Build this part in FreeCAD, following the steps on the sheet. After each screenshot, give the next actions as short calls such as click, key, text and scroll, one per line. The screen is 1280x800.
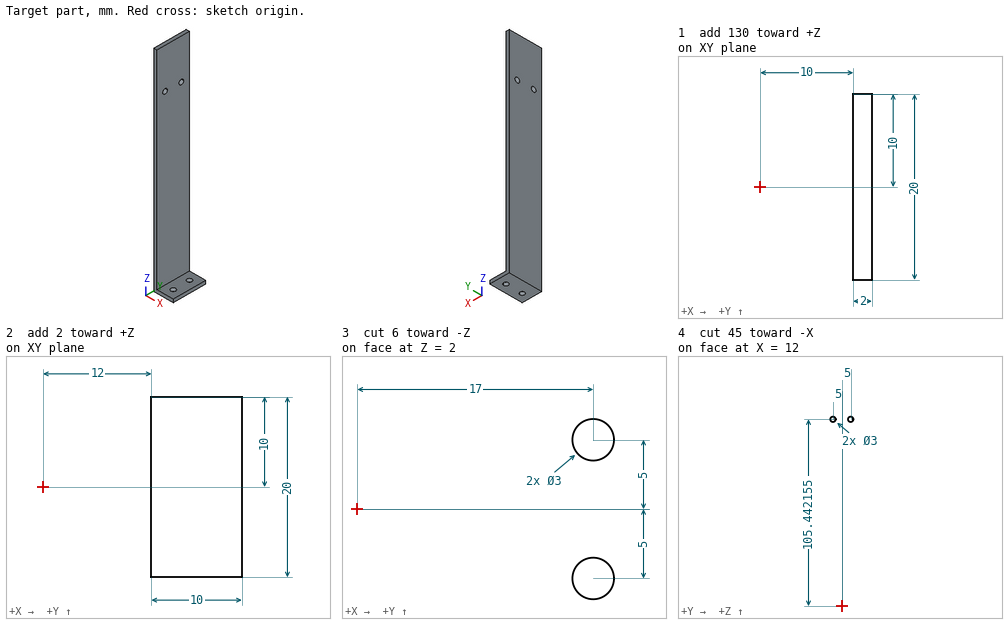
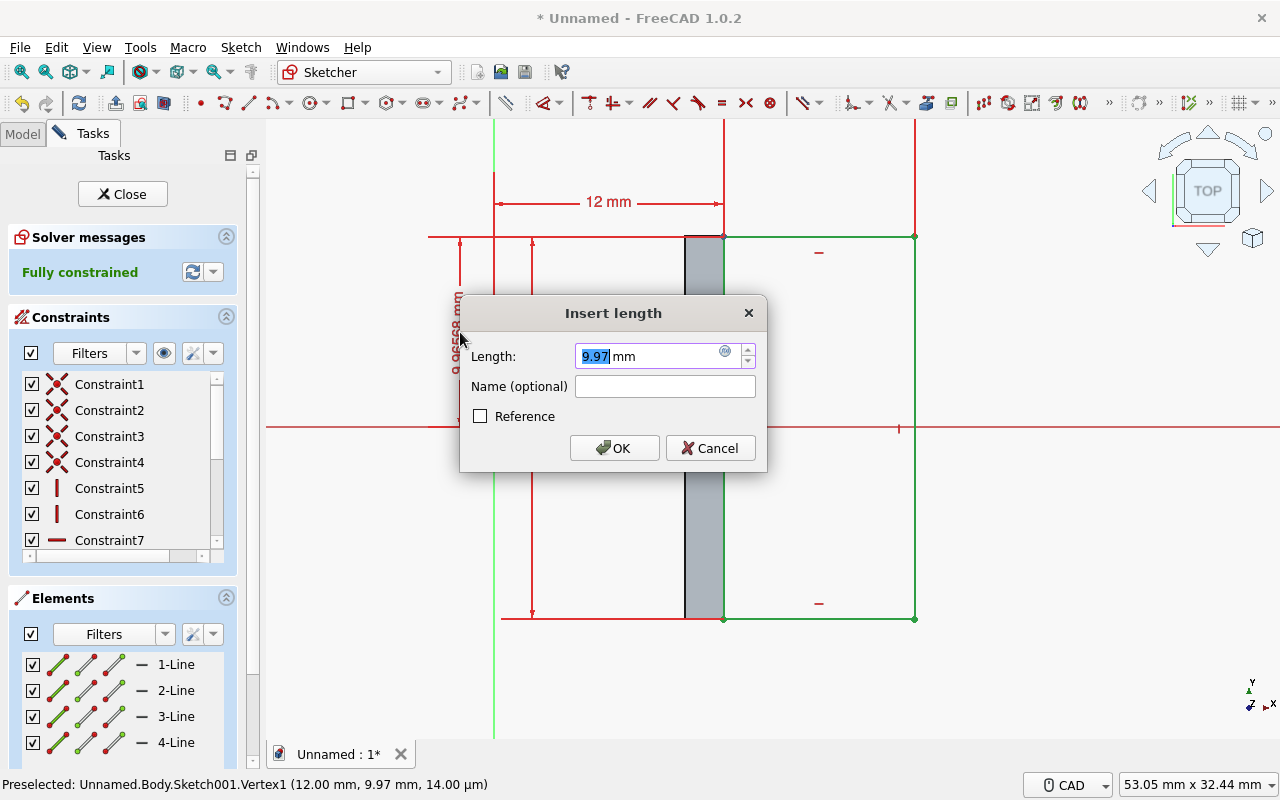
text(10)
key(Return)
key(Escape)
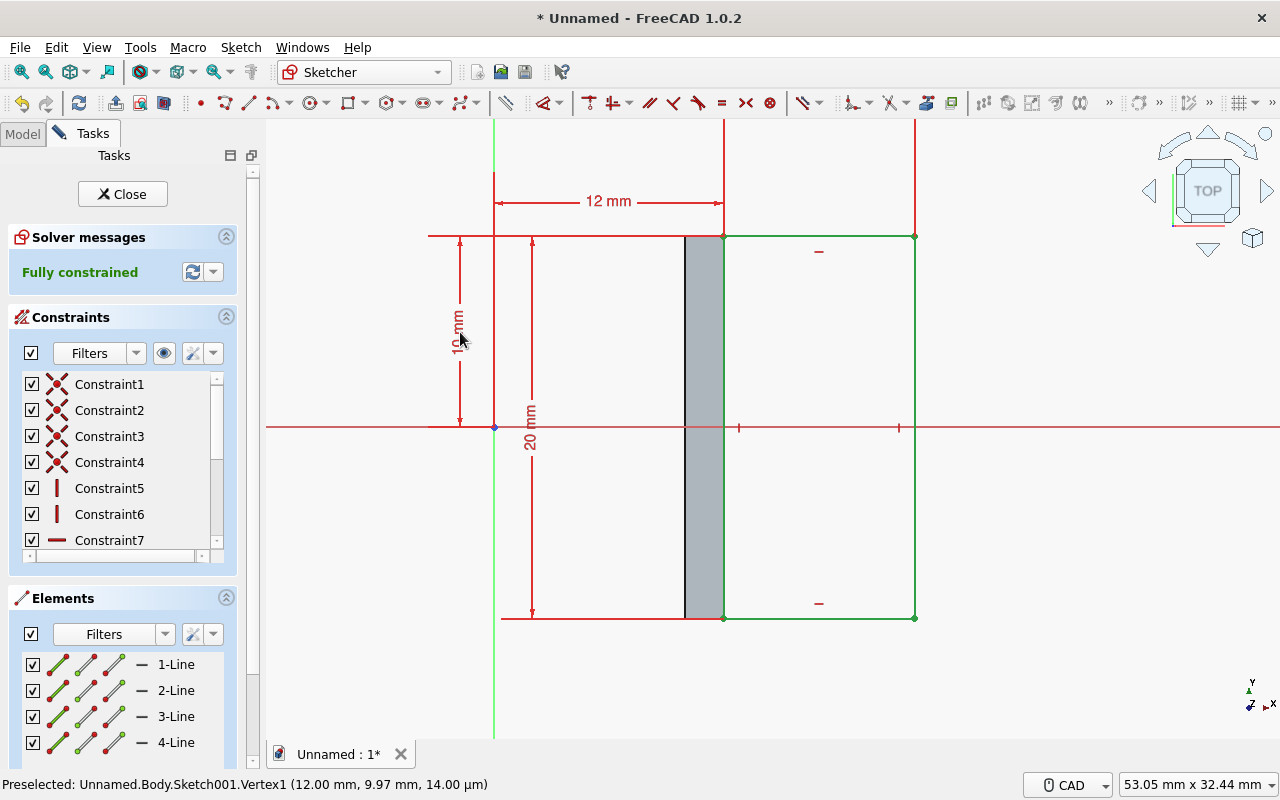
click(123, 194)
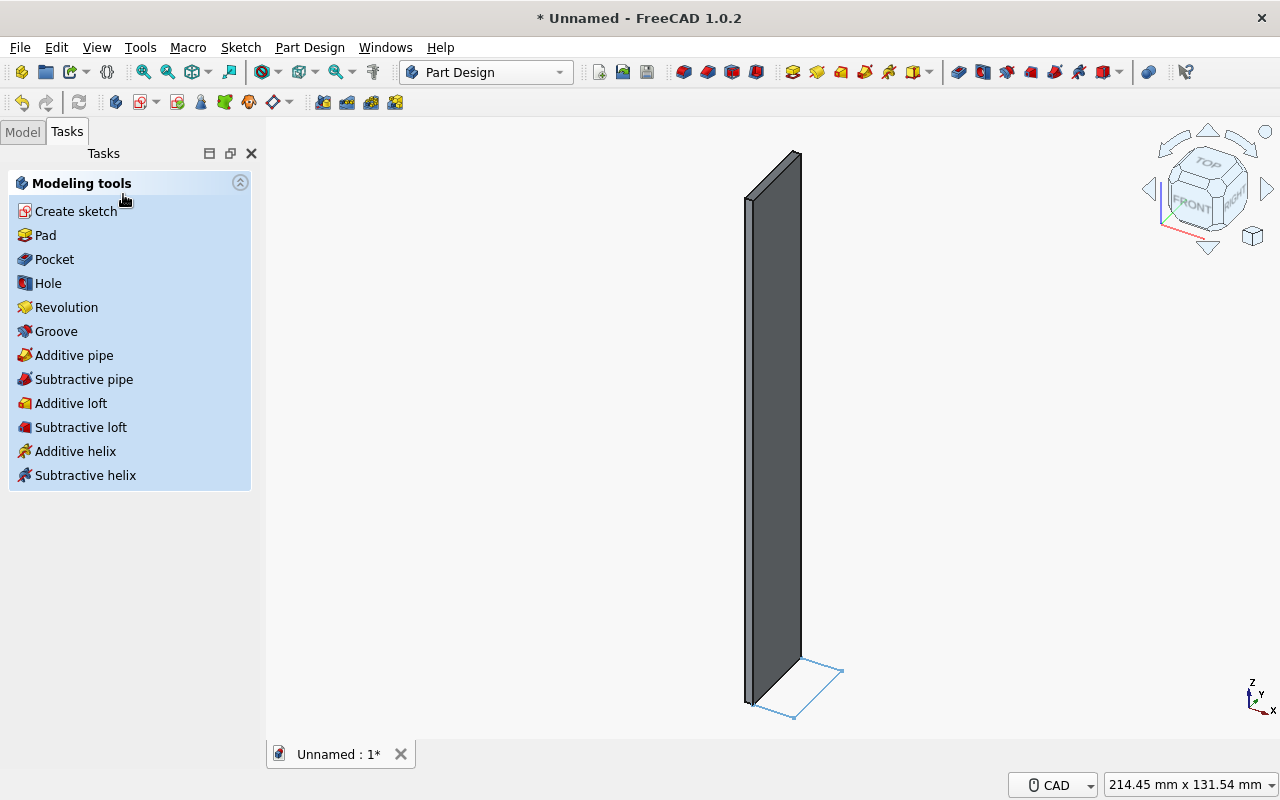
click(794, 72)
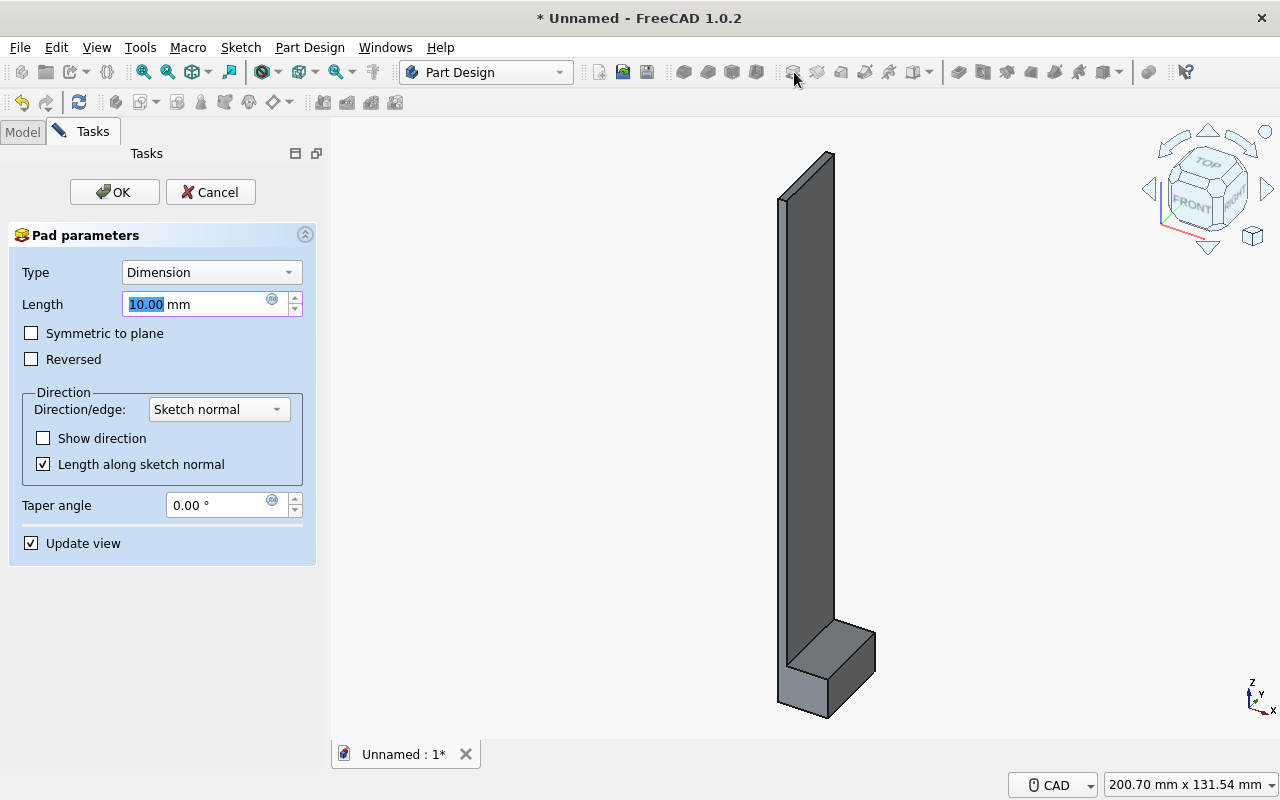
text(2)
key(Tab)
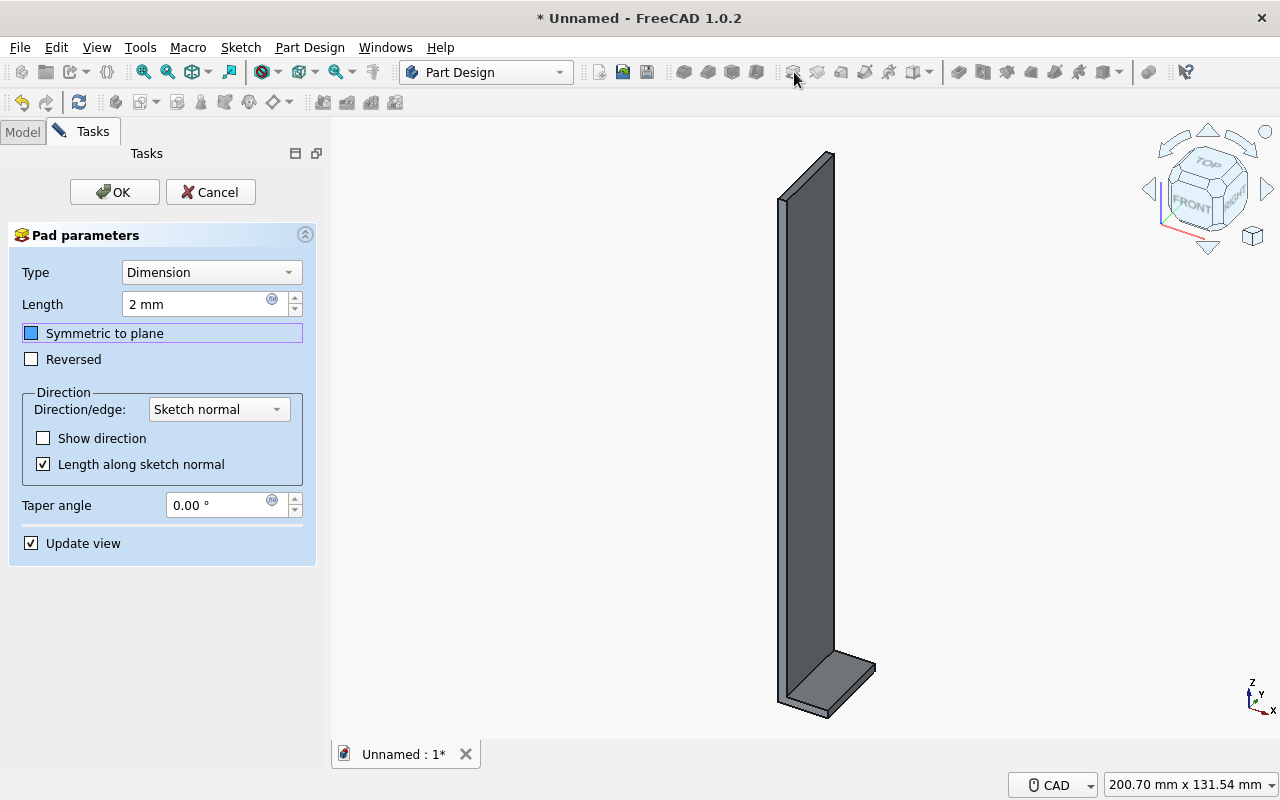
click(115, 192)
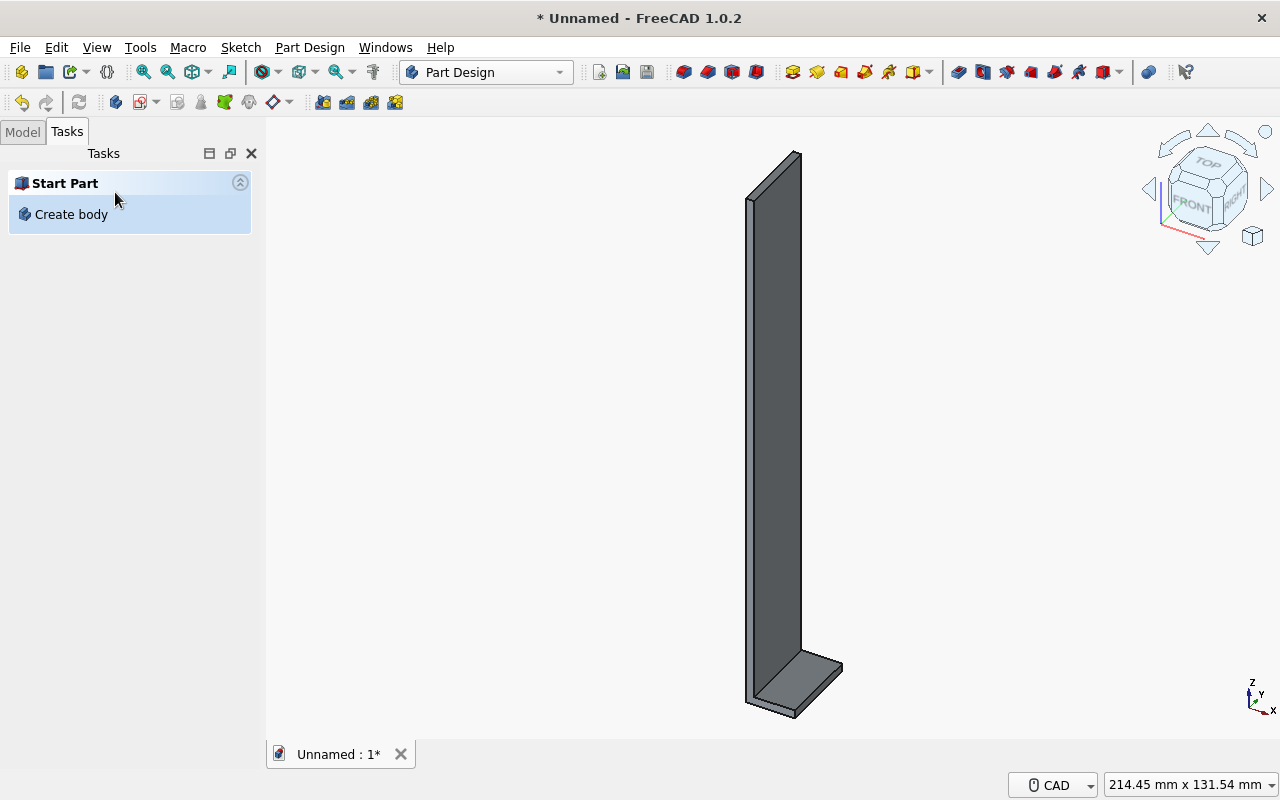
click(805, 673)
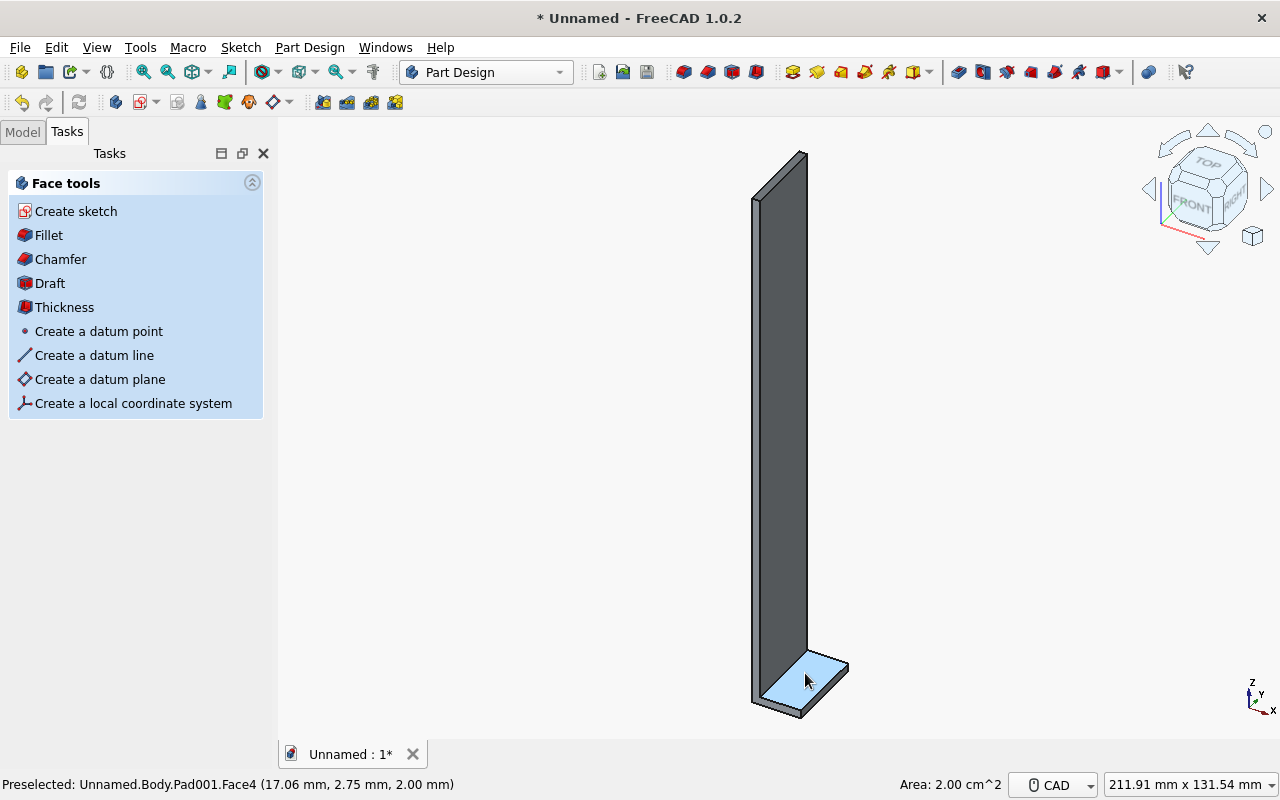
click(140, 102)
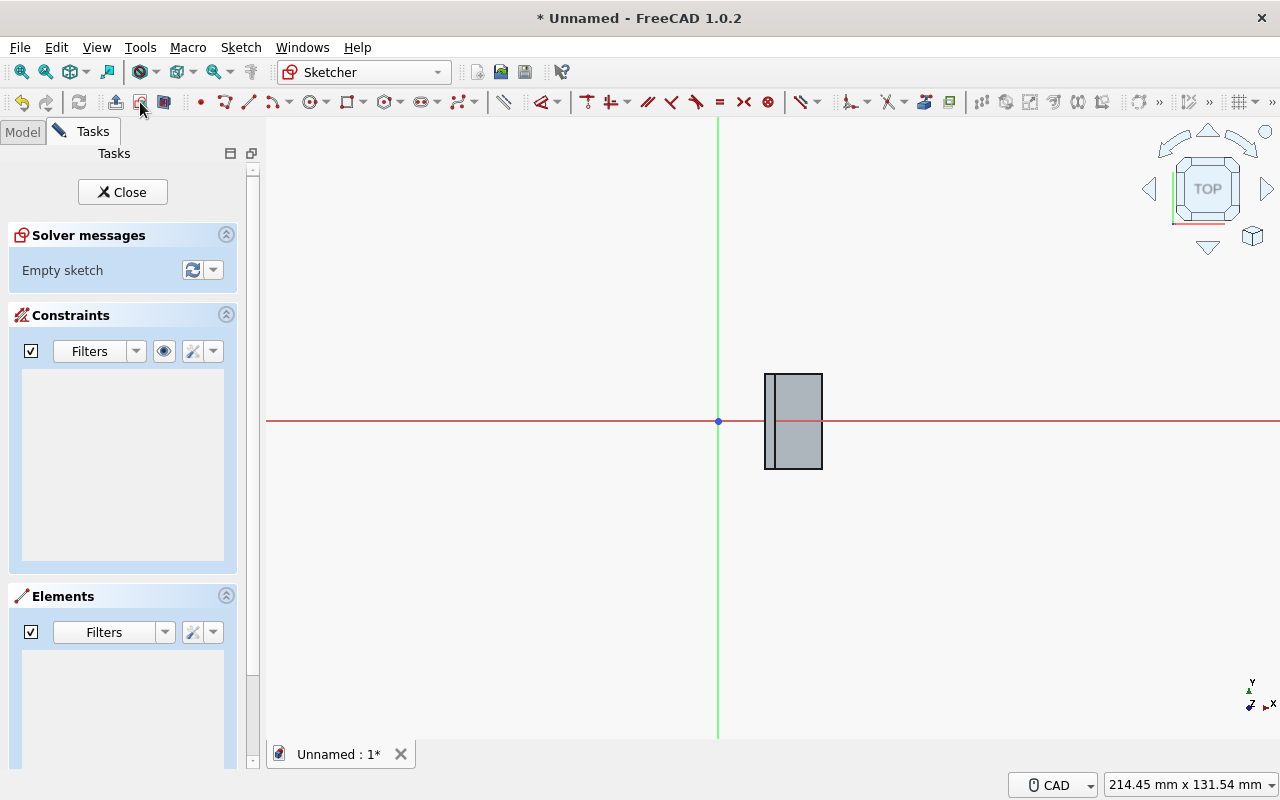
scroll(773, 420, up, 9)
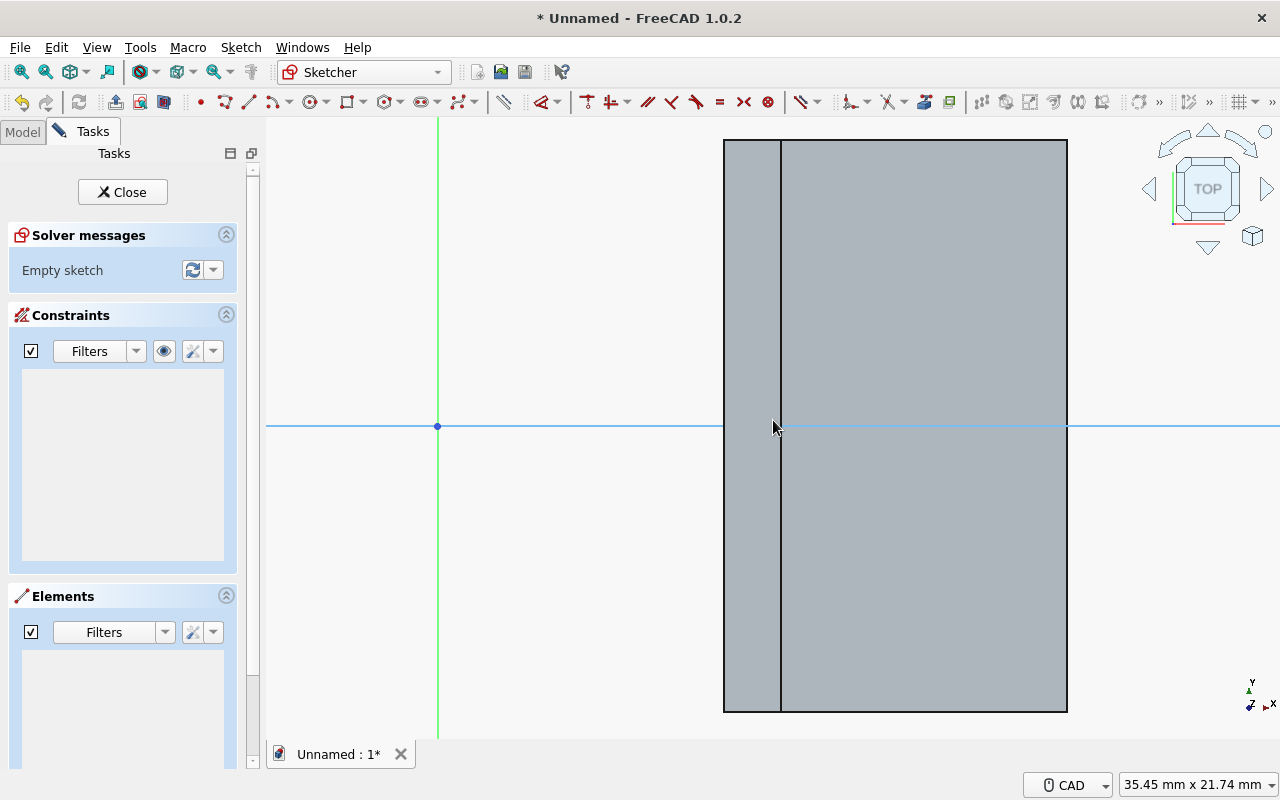
click(310, 102)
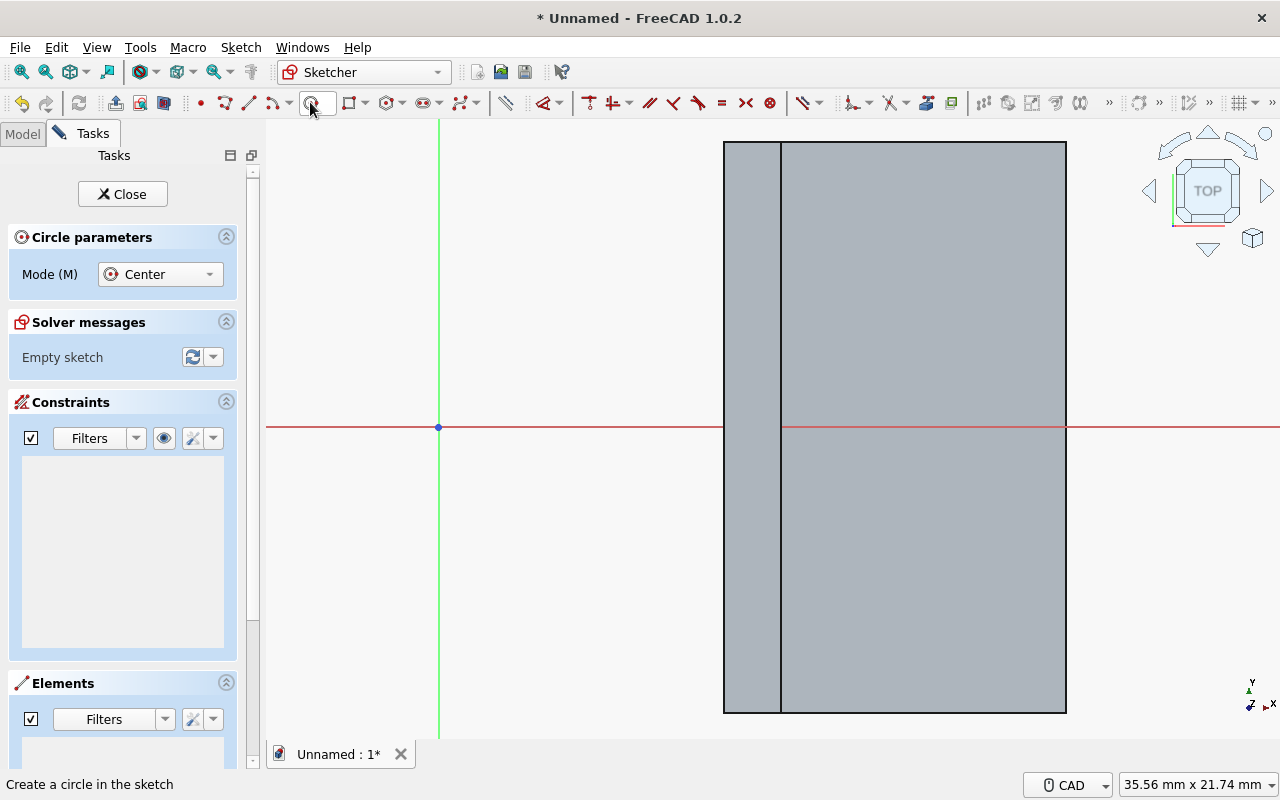
click(924, 285)
move(954, 255)